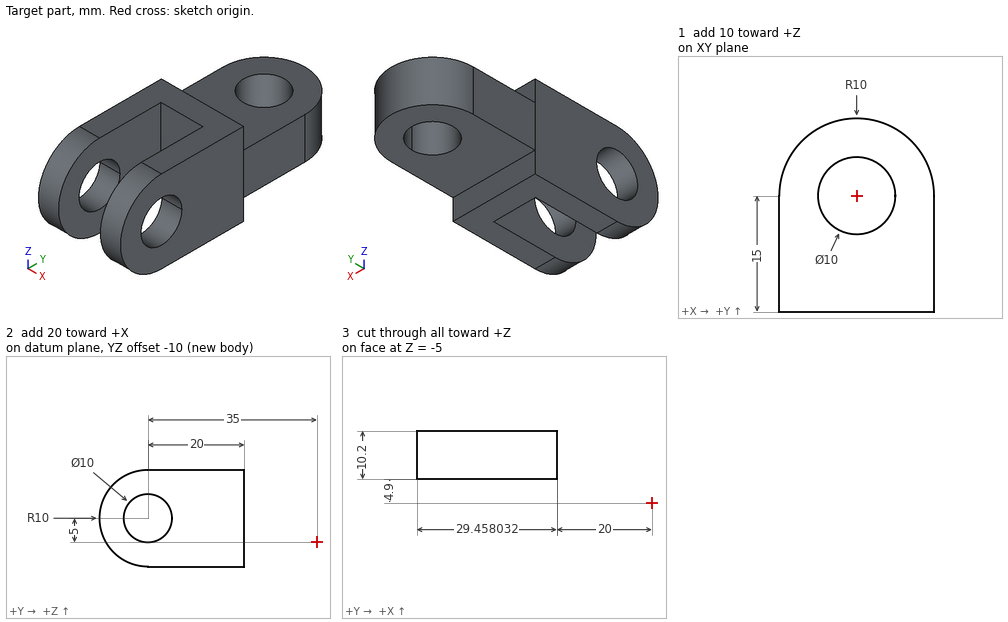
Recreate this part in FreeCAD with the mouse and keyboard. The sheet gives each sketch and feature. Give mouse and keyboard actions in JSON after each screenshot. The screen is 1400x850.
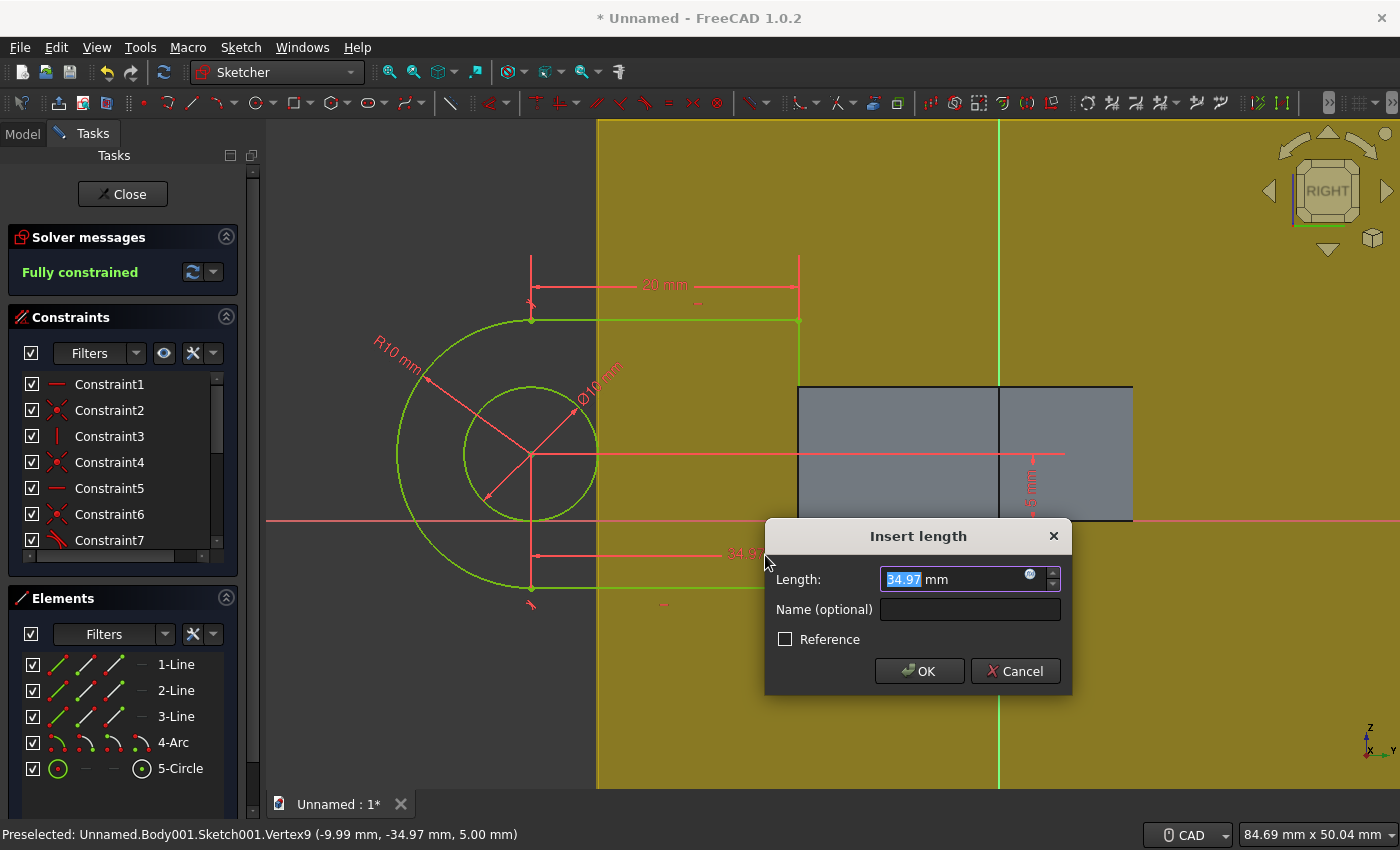
{"action": "type", "text": "35"}
{"action": "key", "text": "Return"}
{"action": "key", "text": "Escape"}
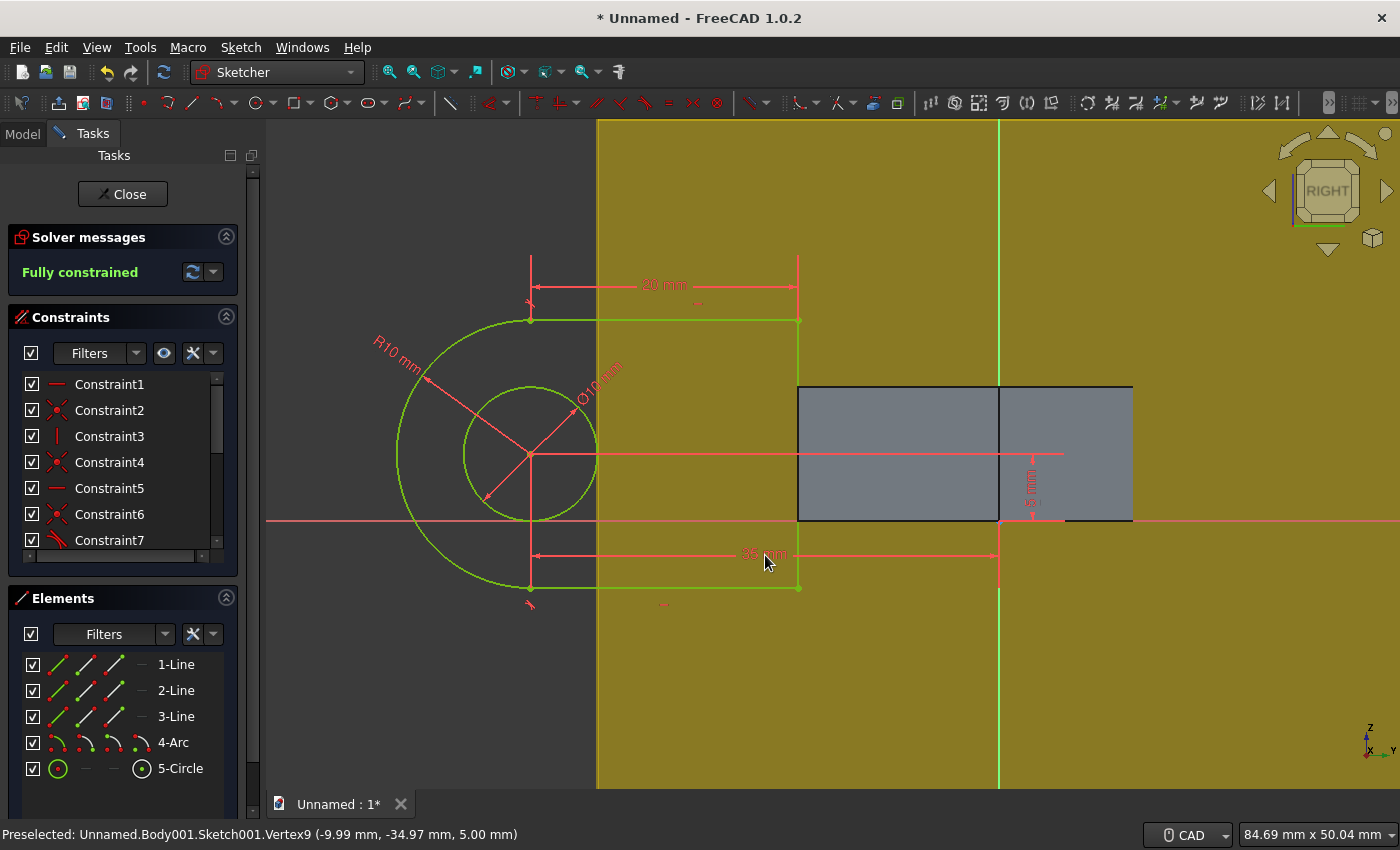
{"action": "left_click", "coordinate": [123, 194]}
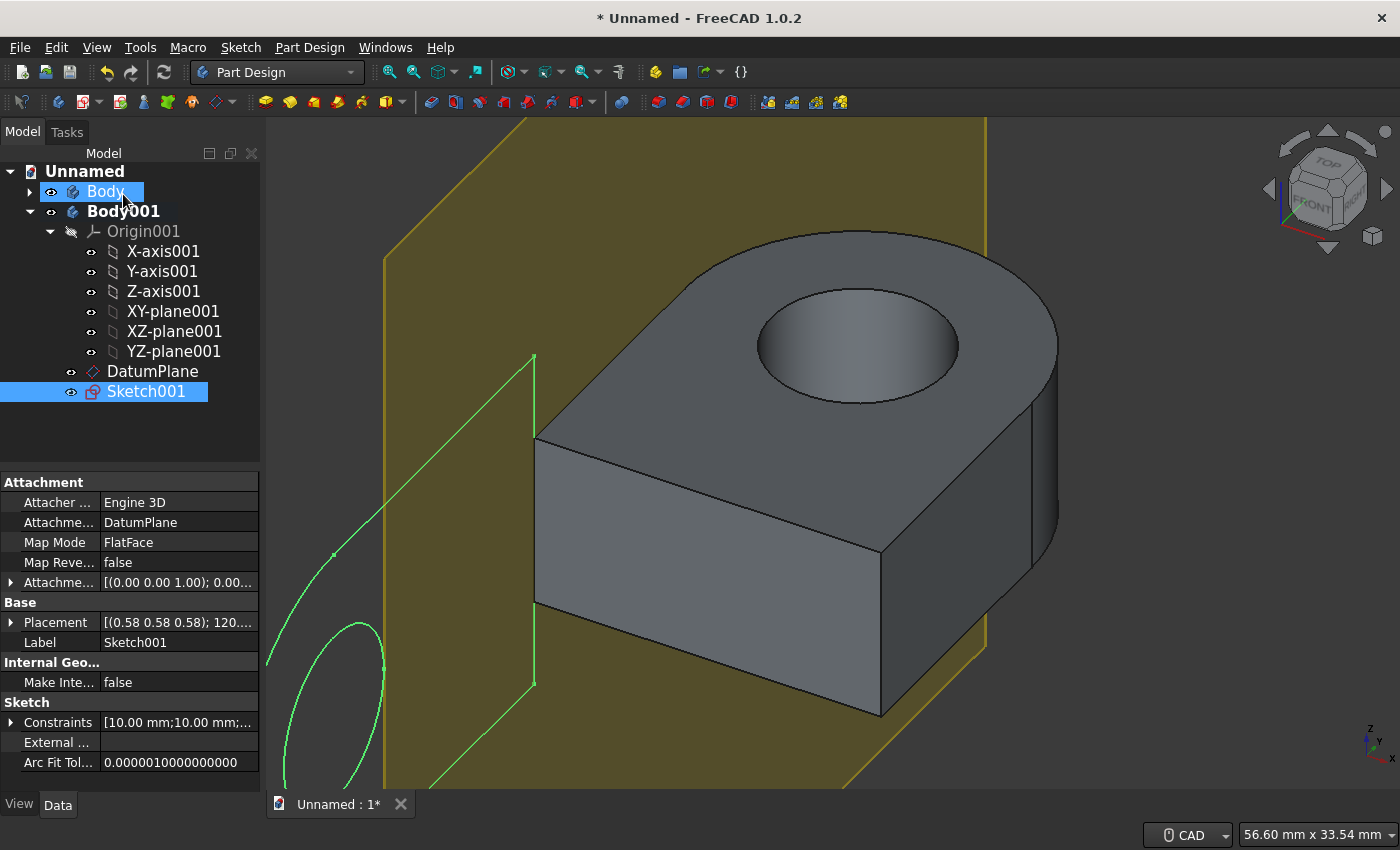
{"action": "left_click", "coordinate": [266, 102]}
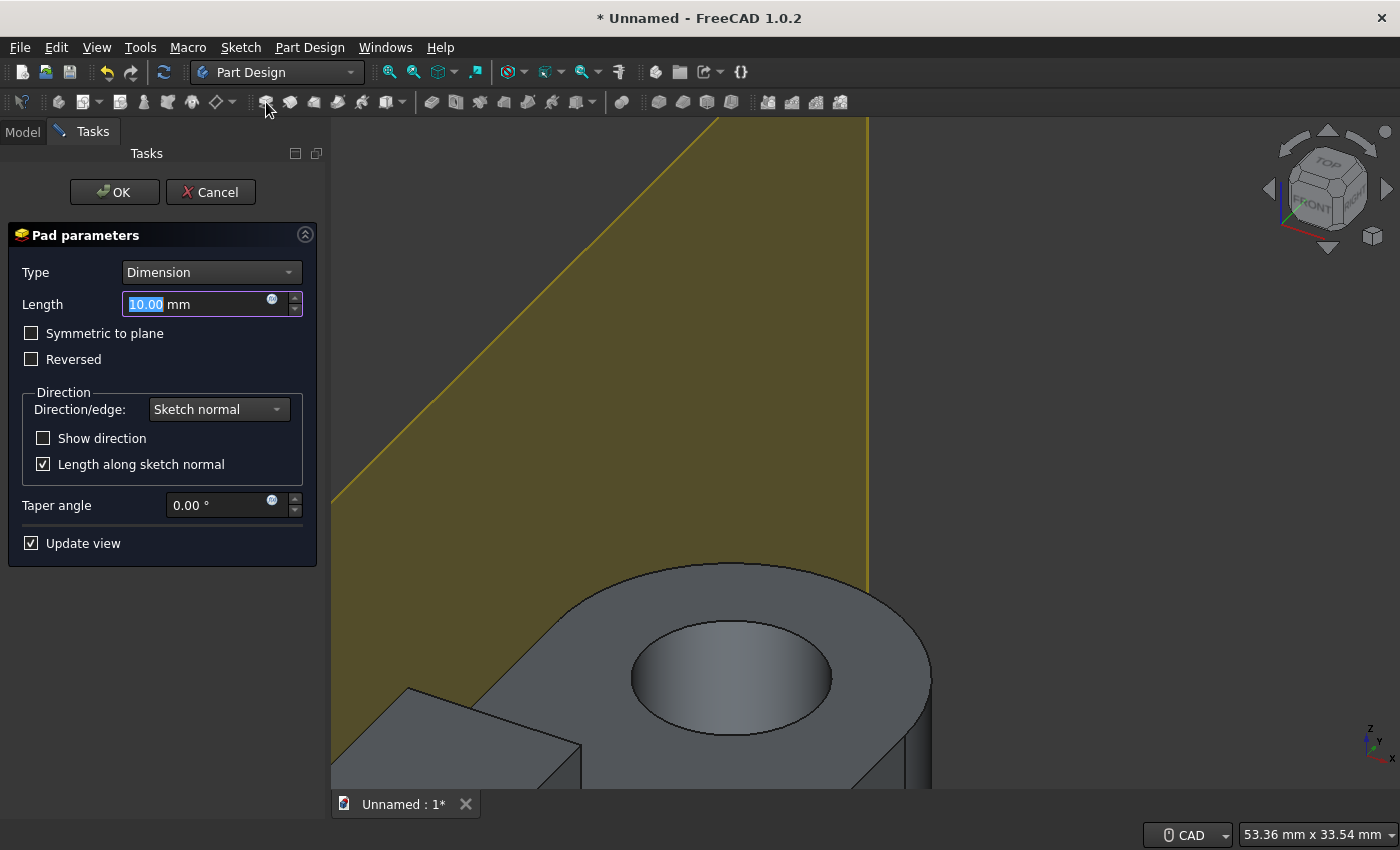
{"action": "type", "text": "20"}
{"action": "key", "text": "Tab"}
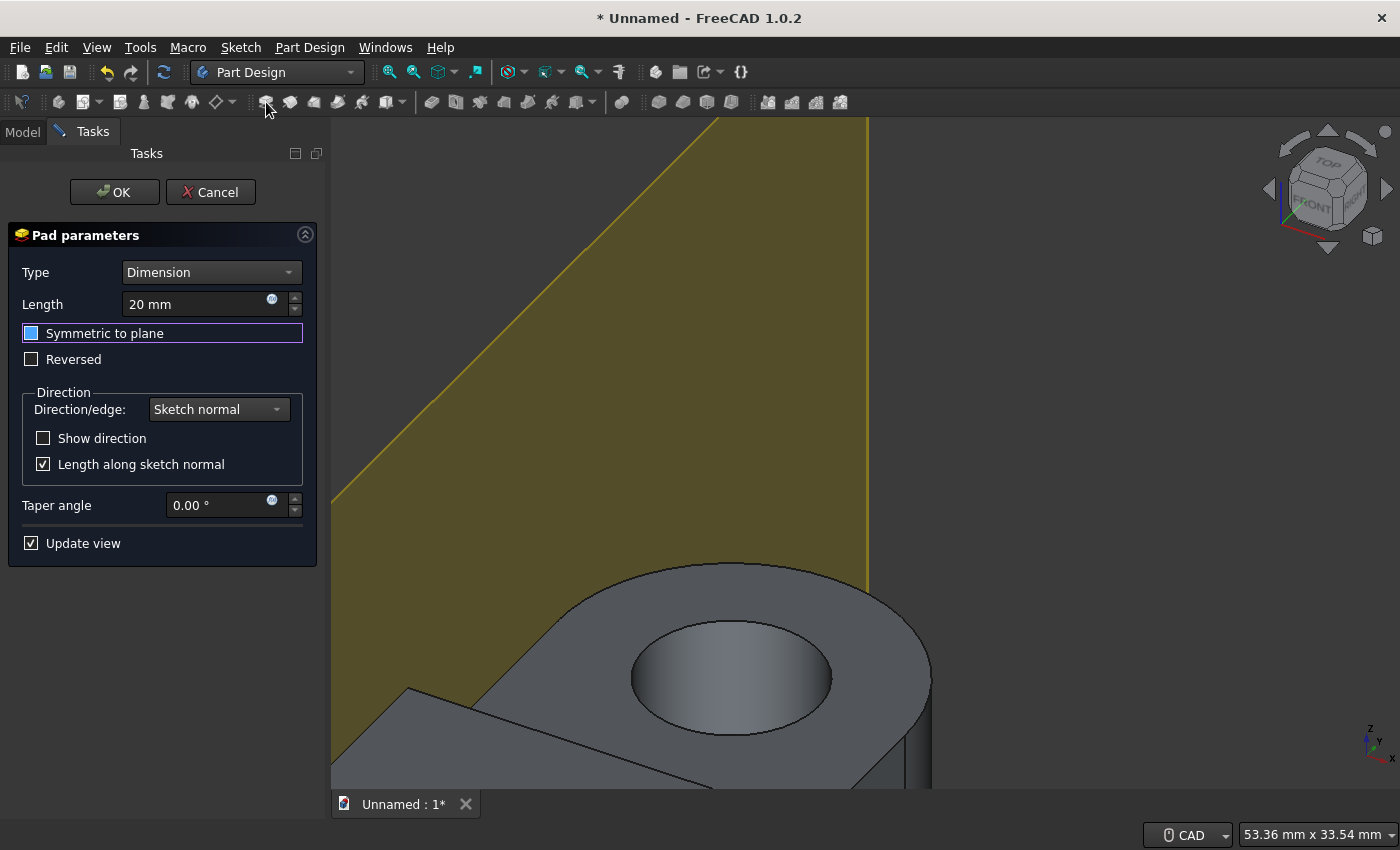
{"action": "left_click", "coordinate": [115, 192]}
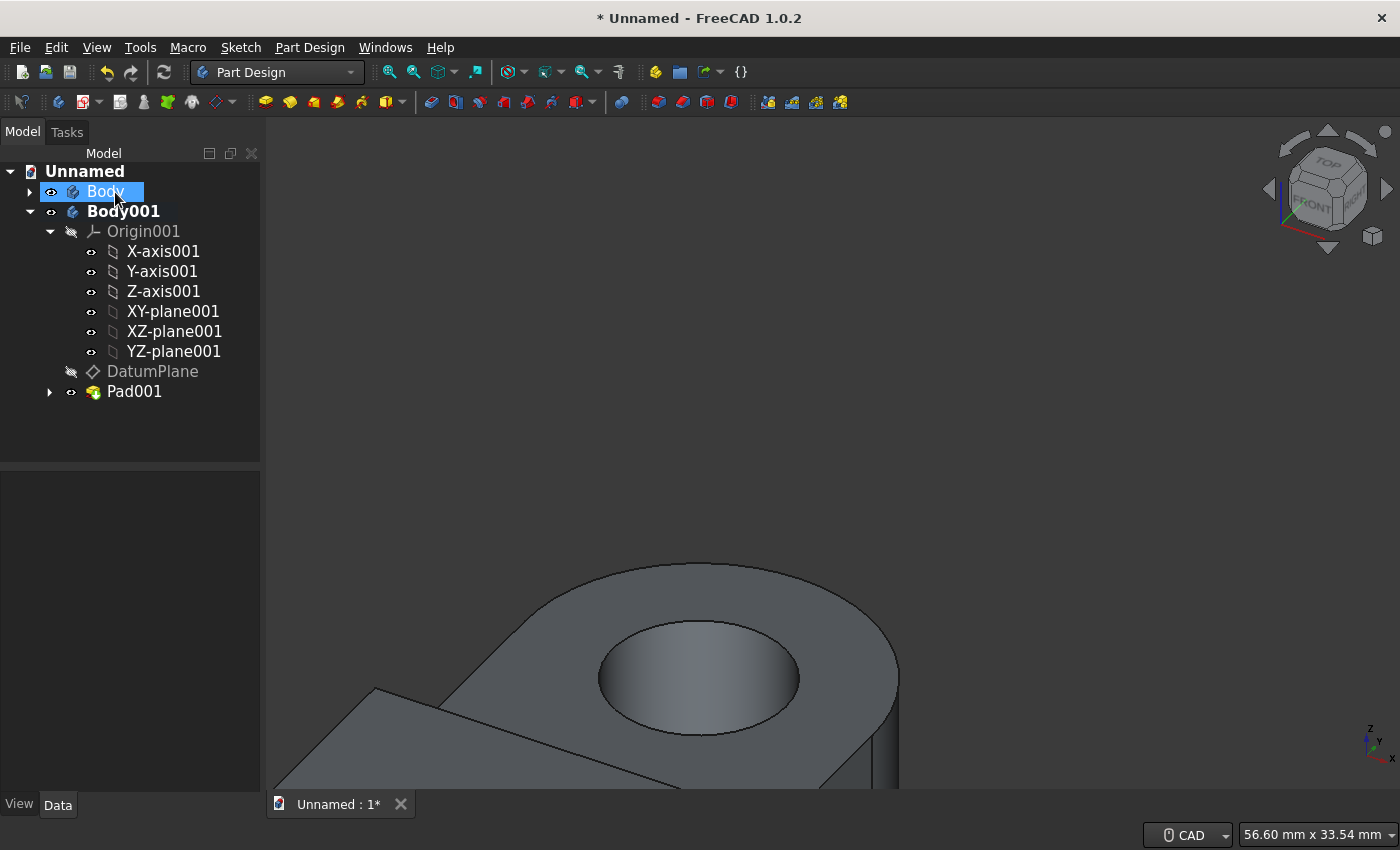
{"action": "left_click", "coordinate": [390, 72]}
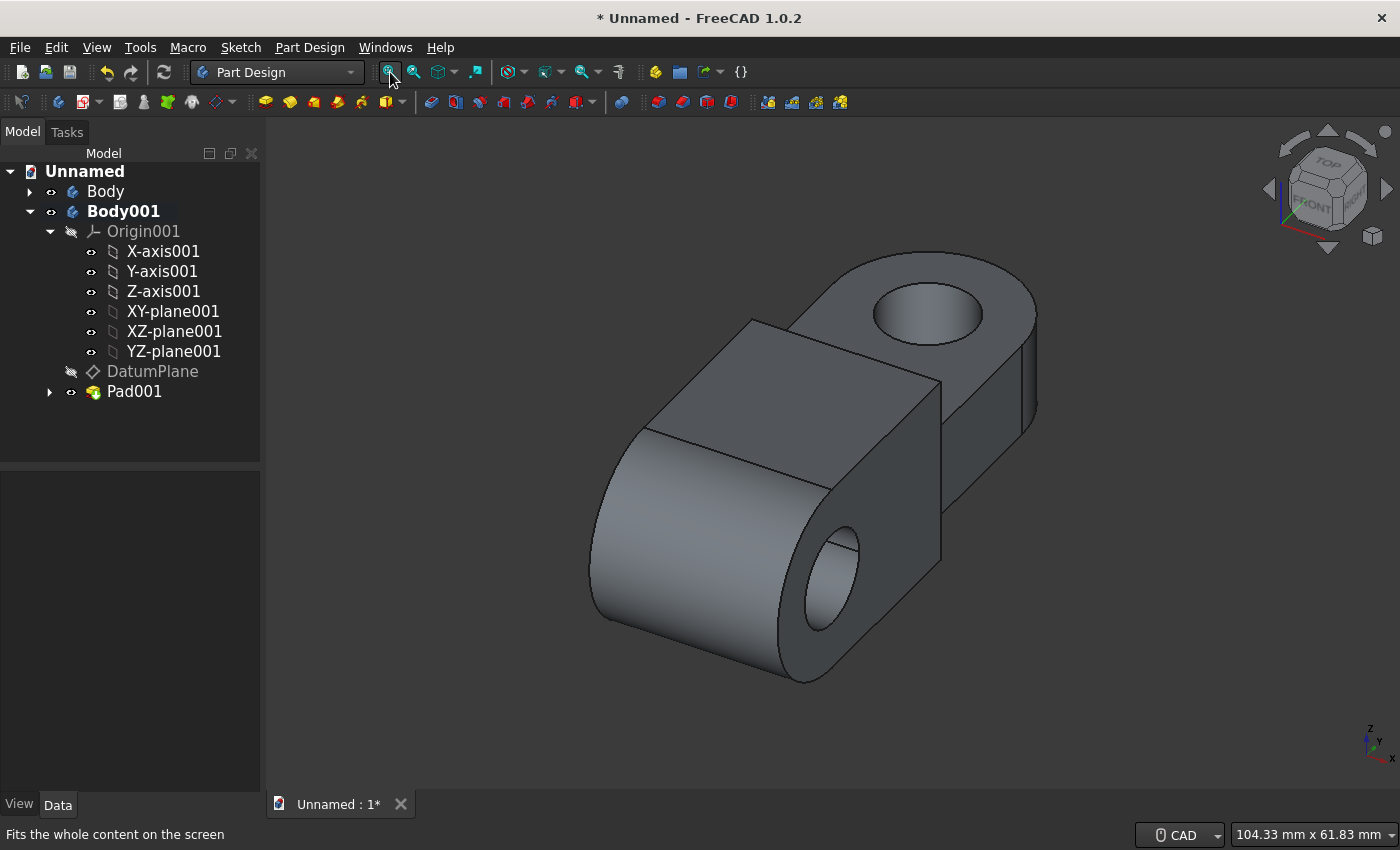
{"action": "key", "text": "5"}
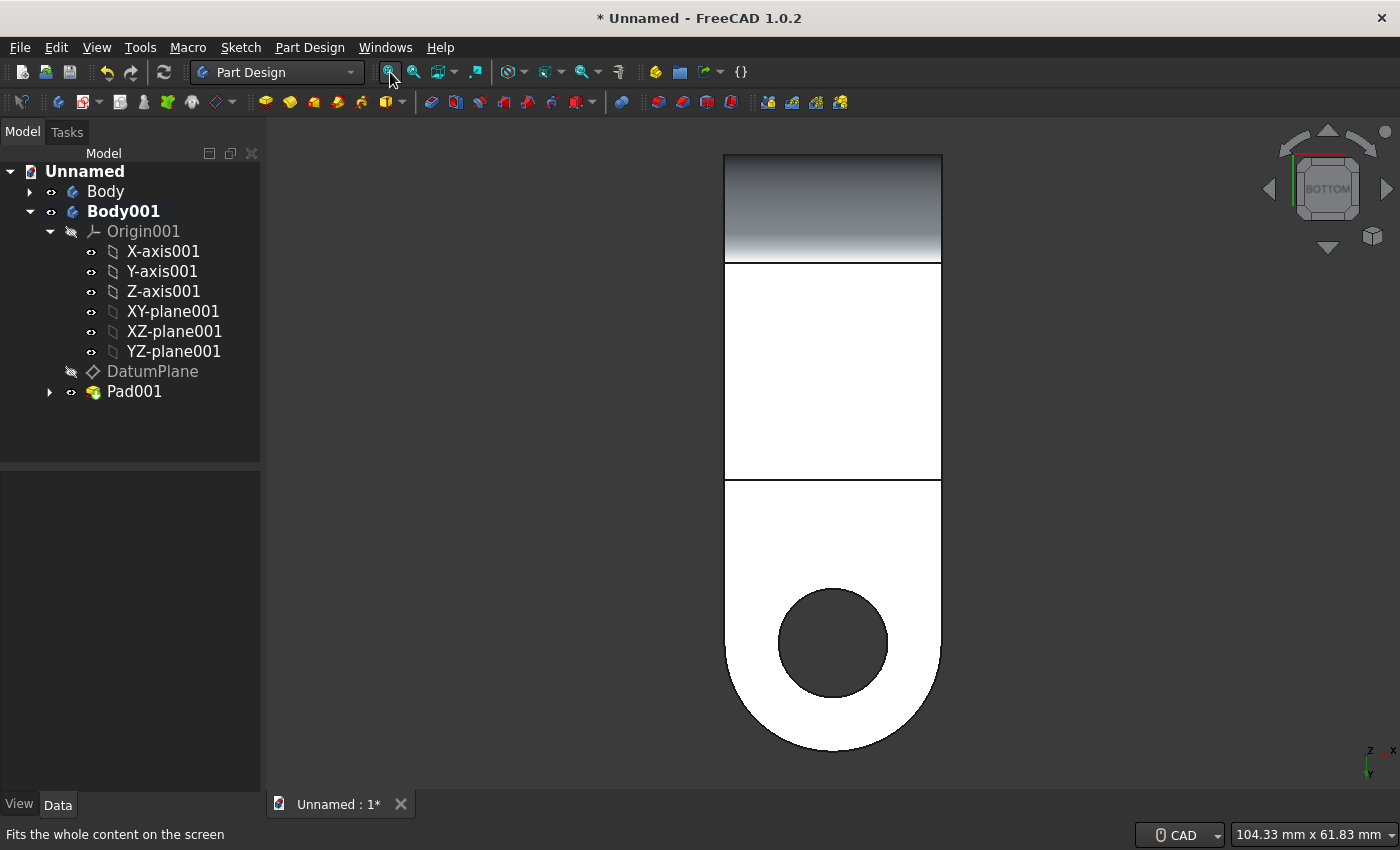
{"action": "left_click", "coordinate": [833, 370]}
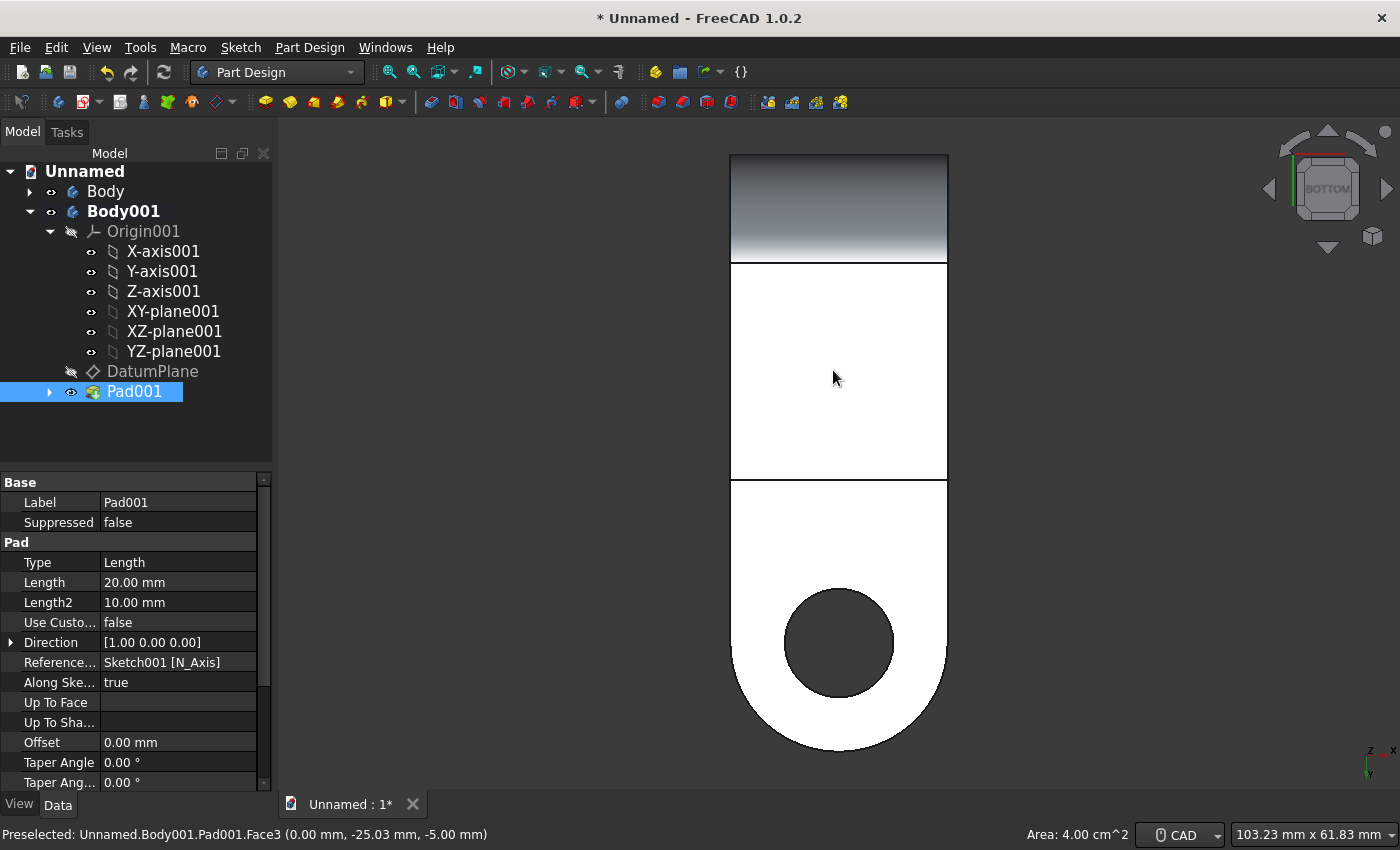
{"action": "left_click", "coordinate": [84, 102]}